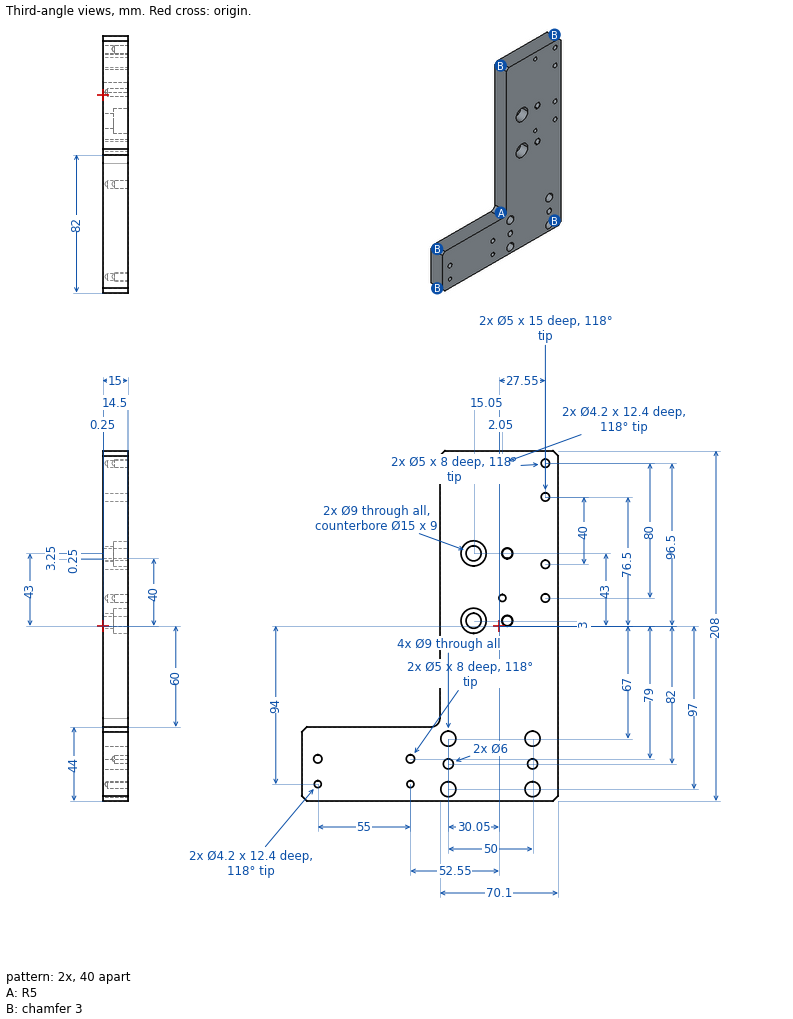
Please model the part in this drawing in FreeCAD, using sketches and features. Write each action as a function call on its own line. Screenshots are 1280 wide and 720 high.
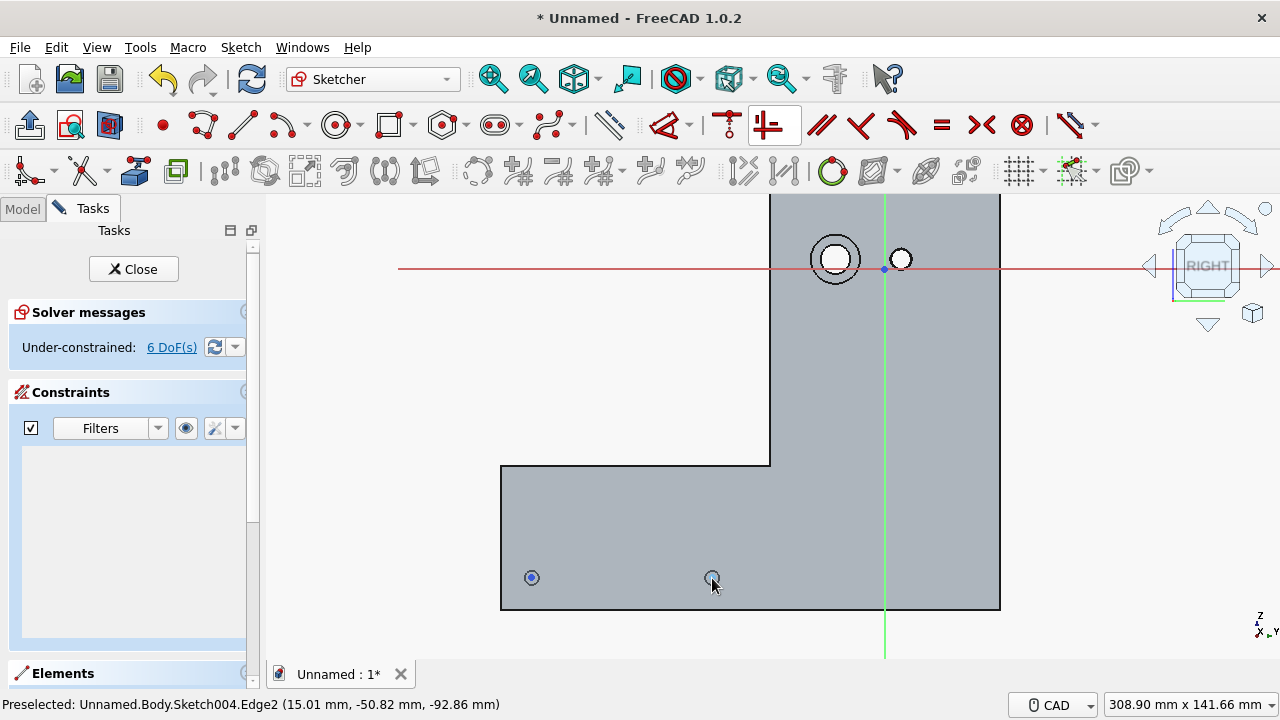
scroll(537, 573, up, 4)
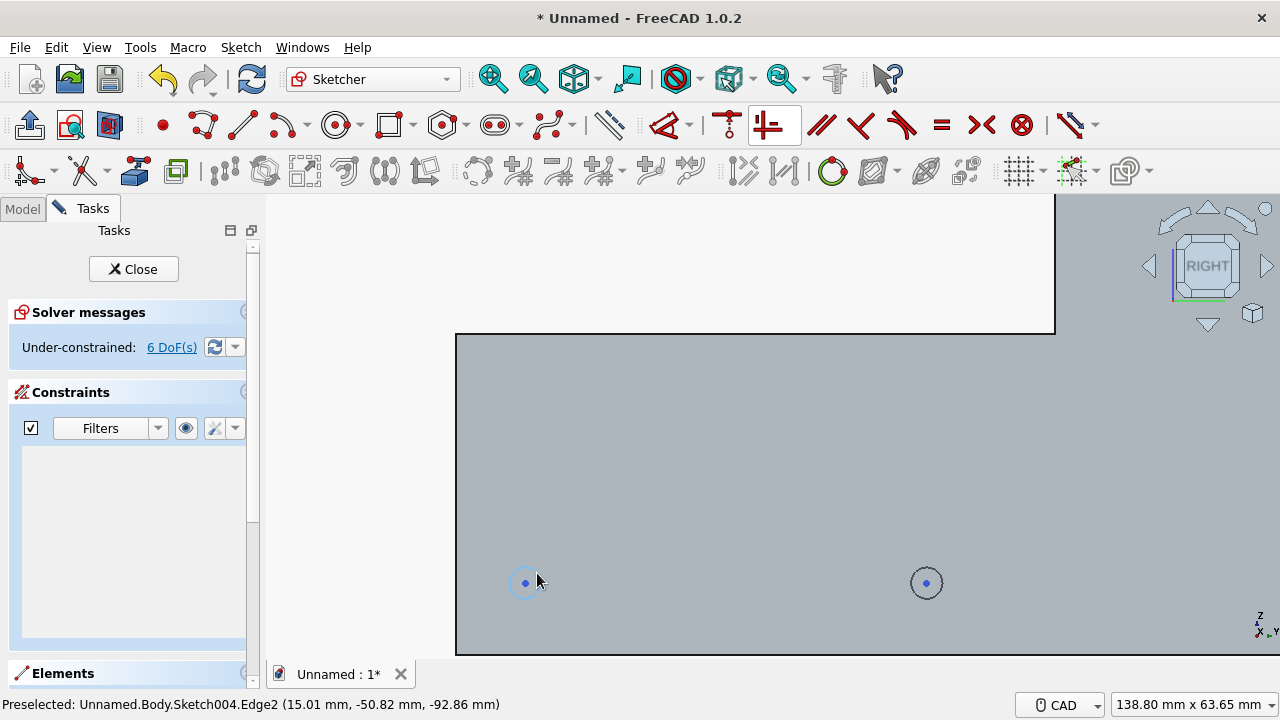
click(536, 572)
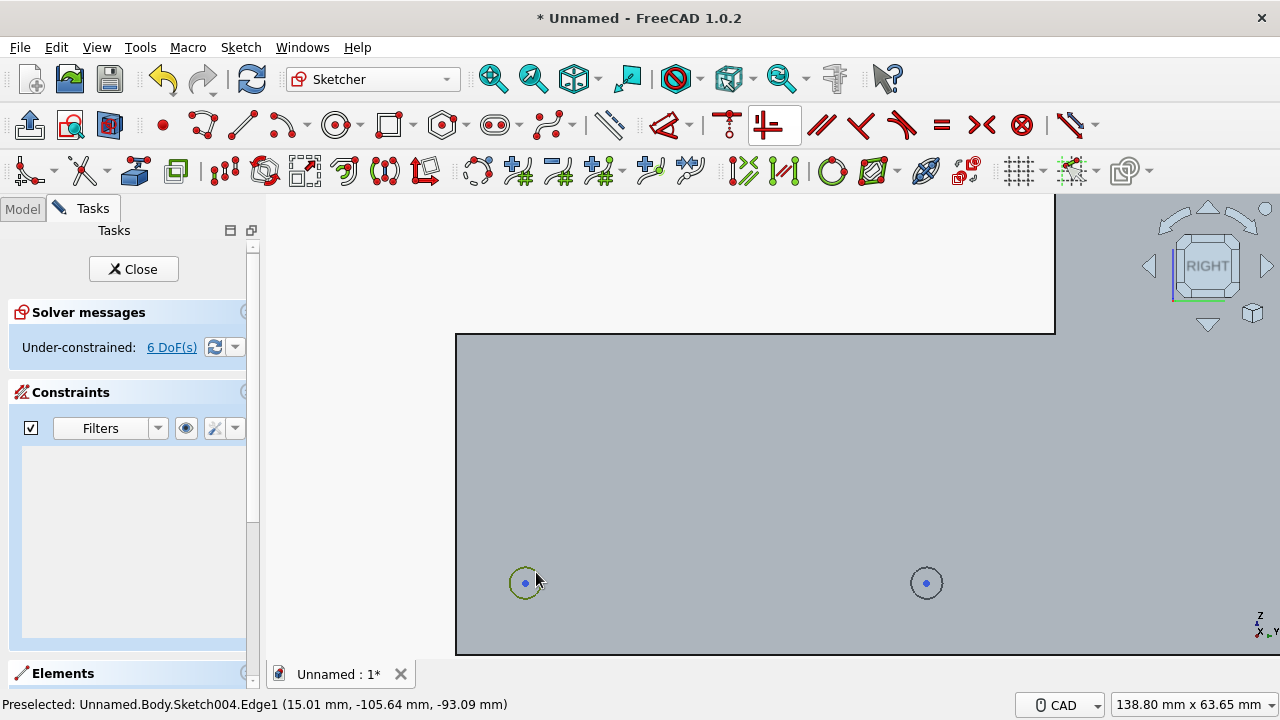
click(938, 572)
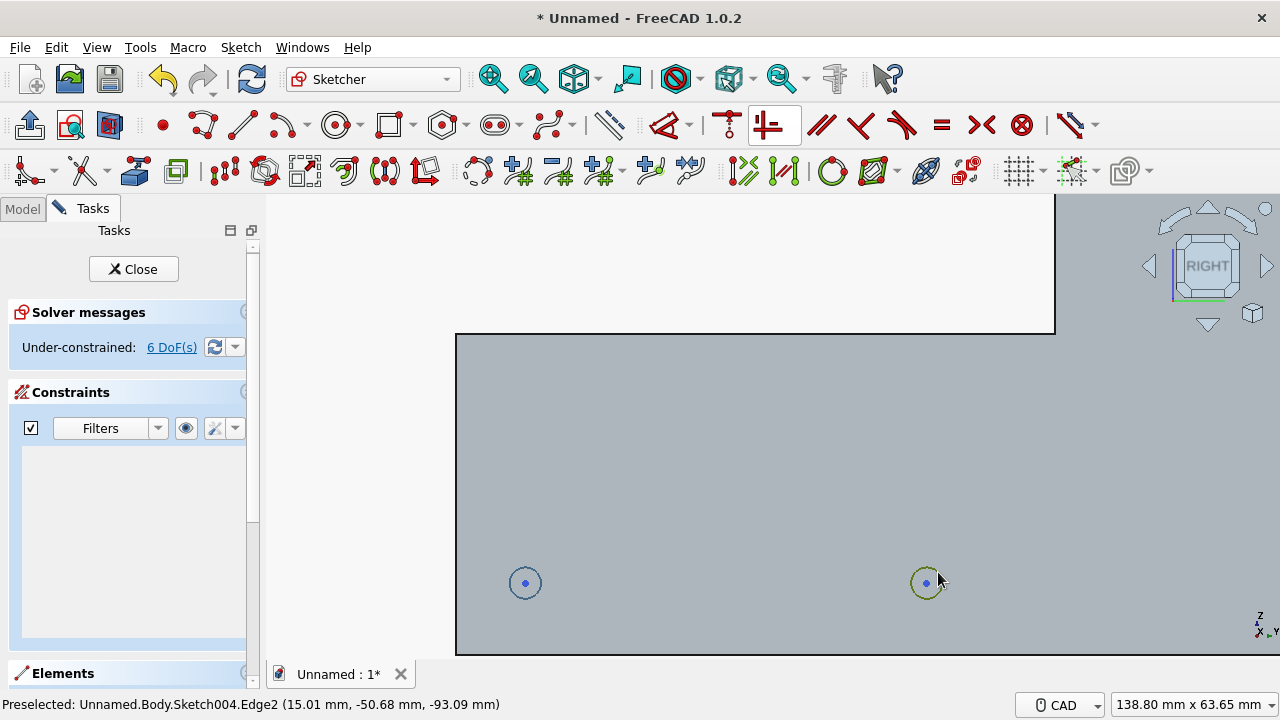
key(e)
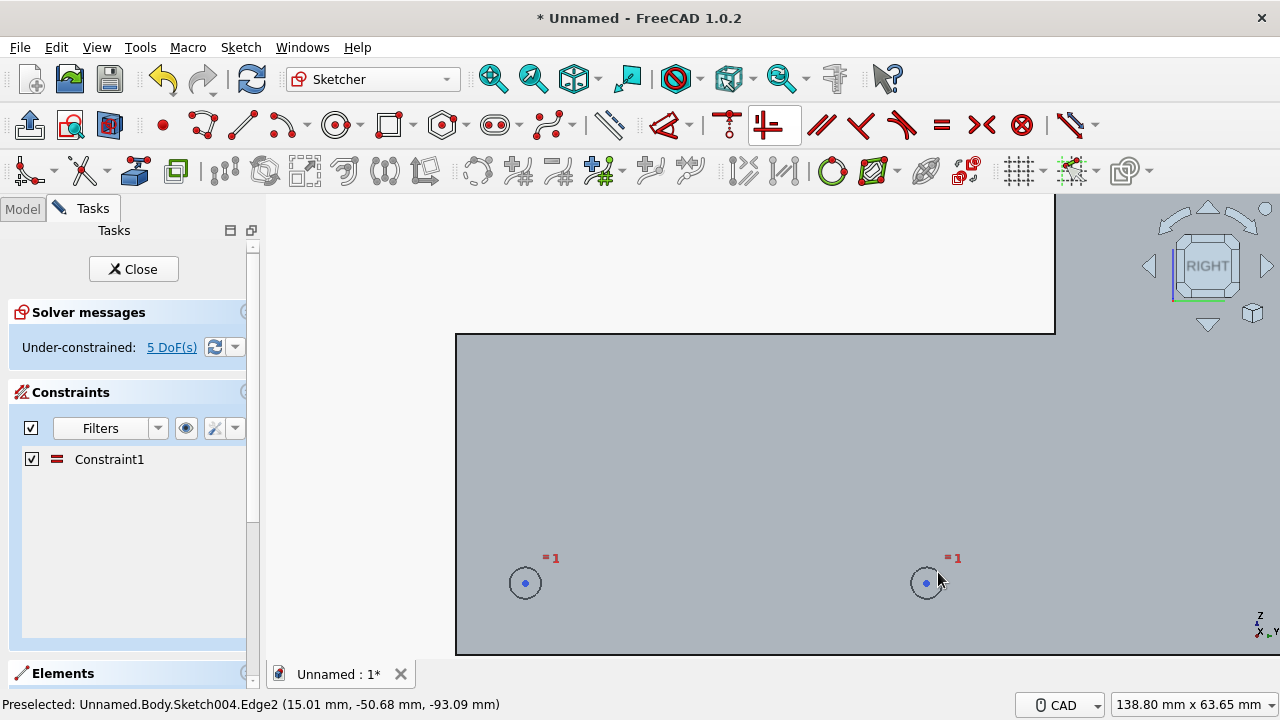
click(525, 583)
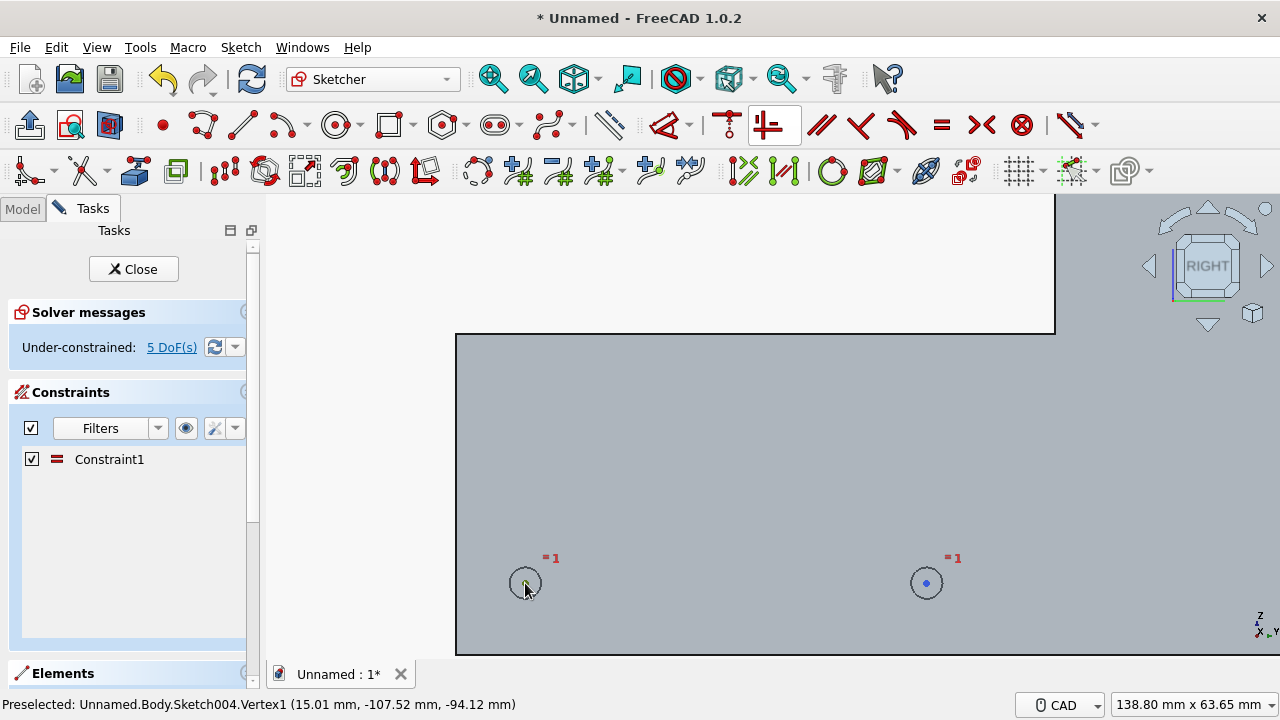
click(927, 583)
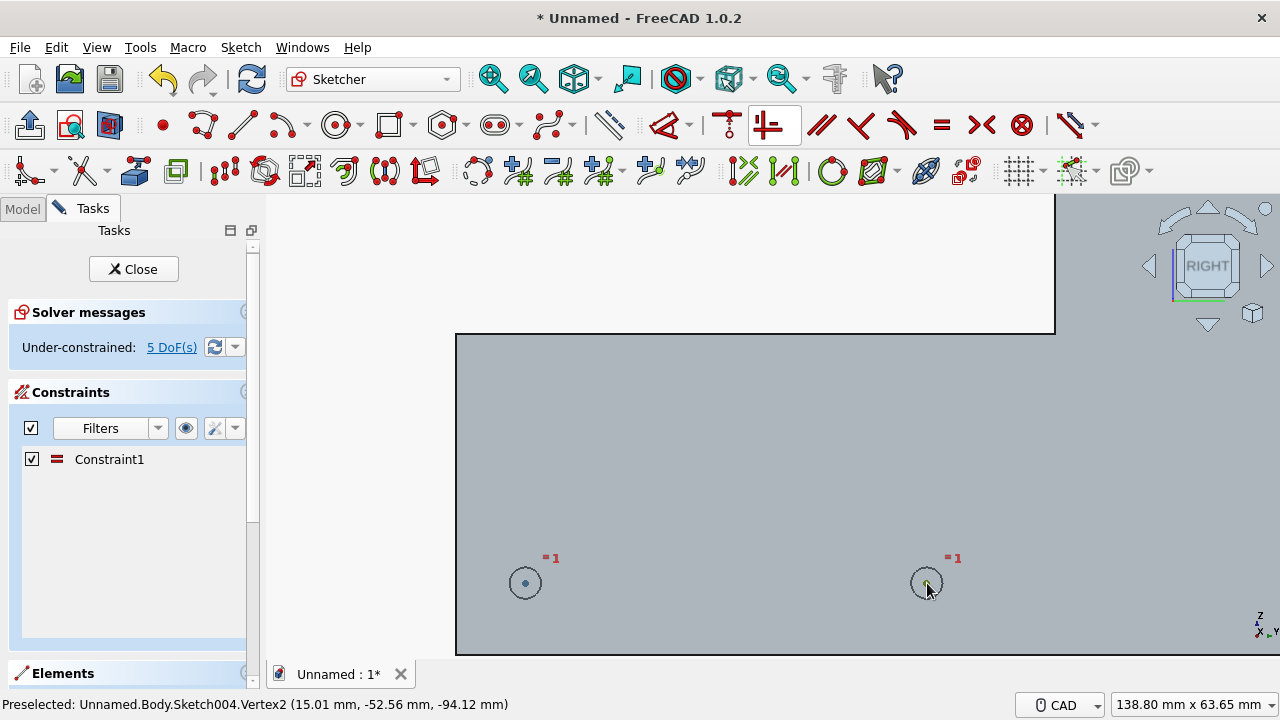
click(796, 126)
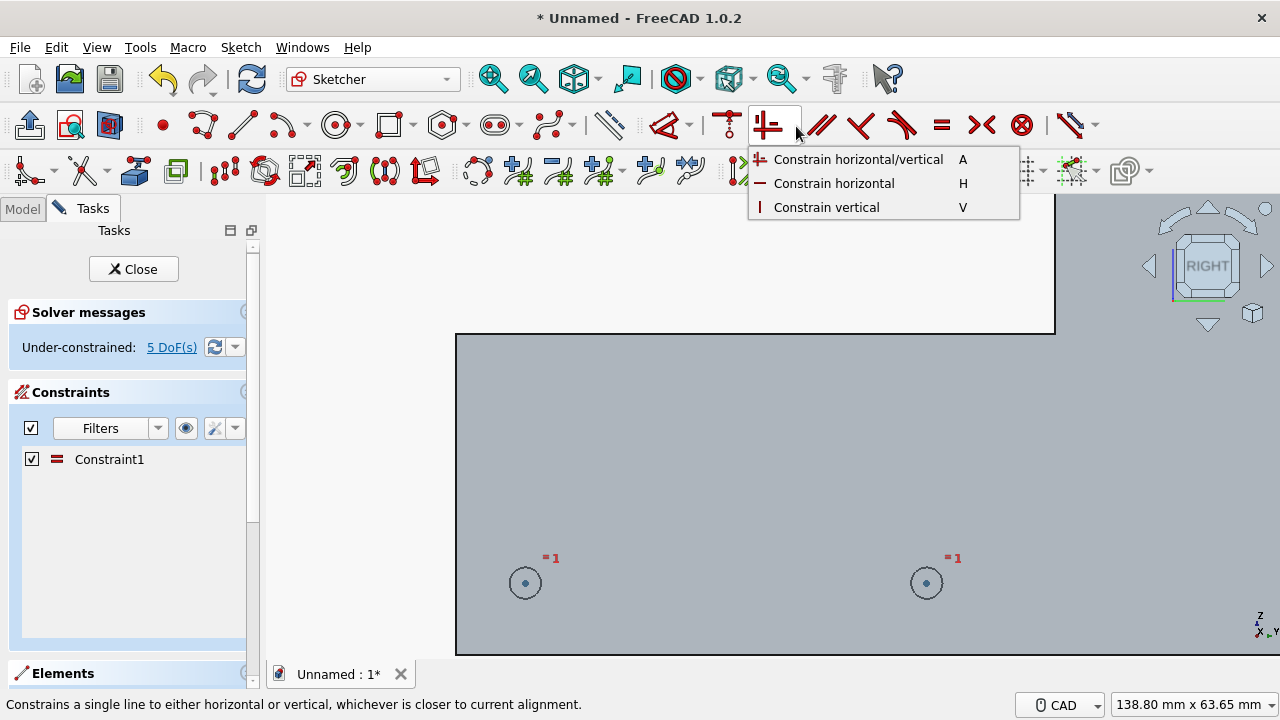
click(884, 183)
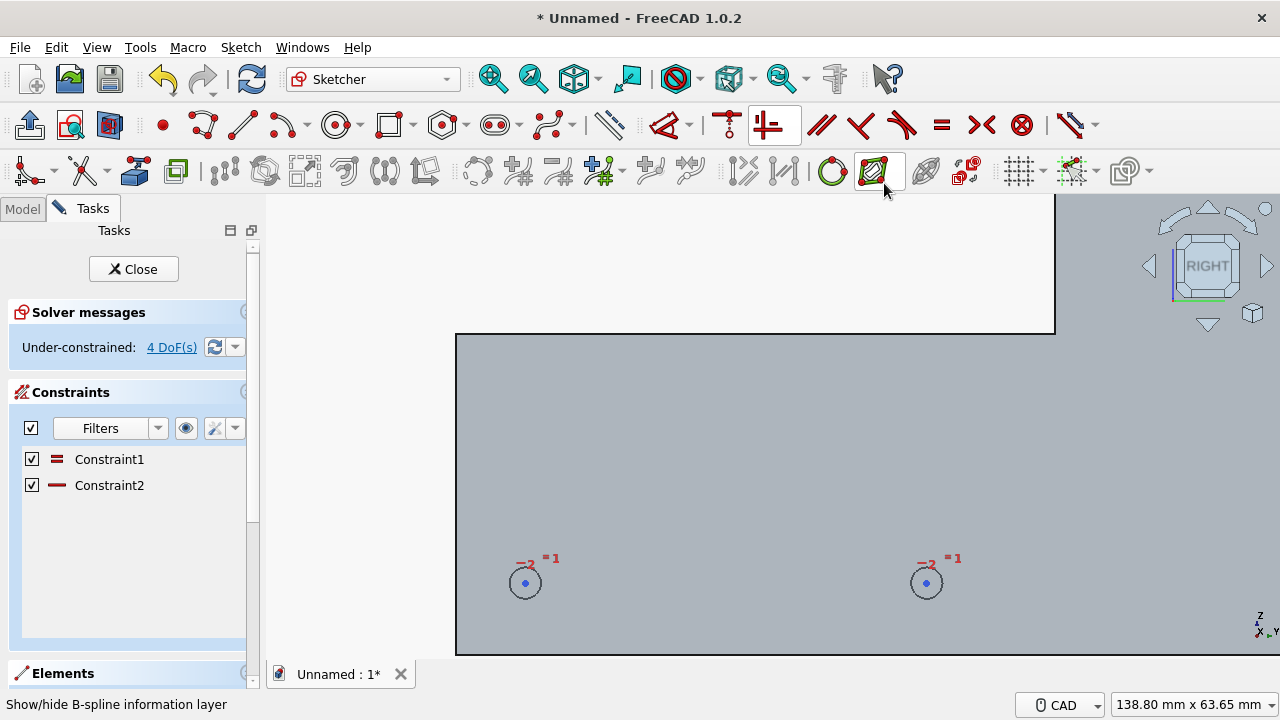
key(d)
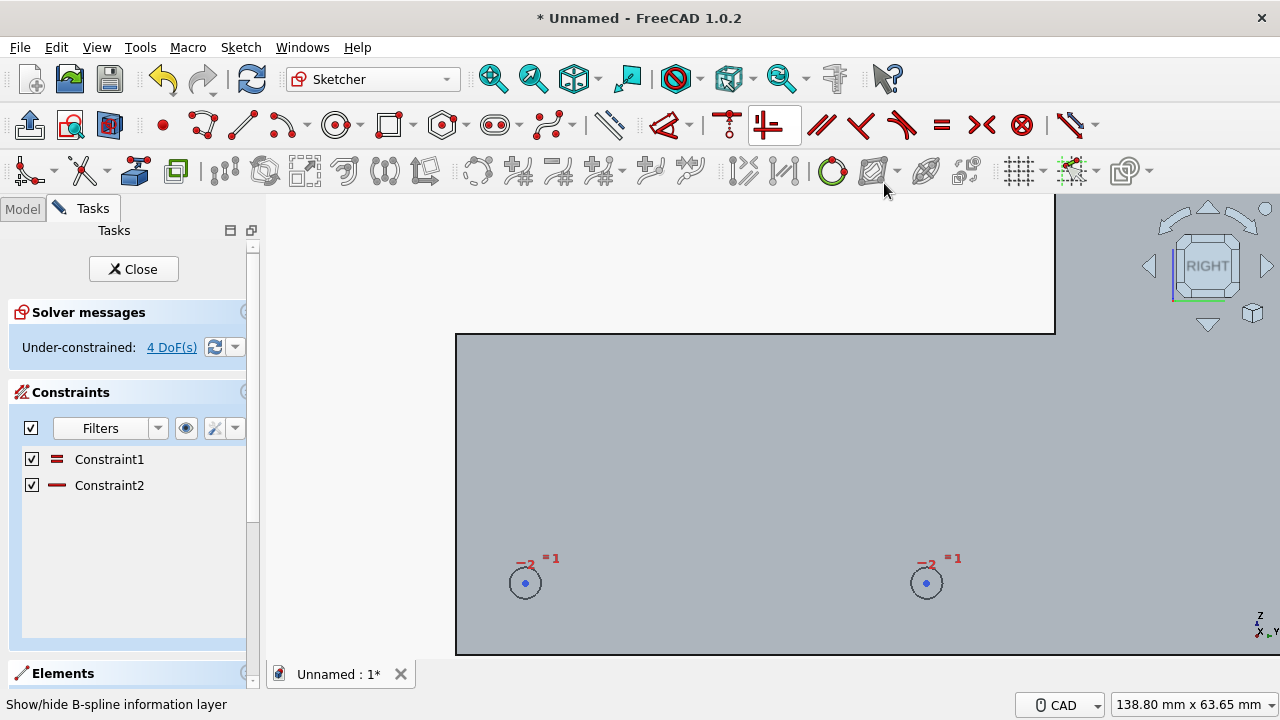
scroll(536, 572, up, 2)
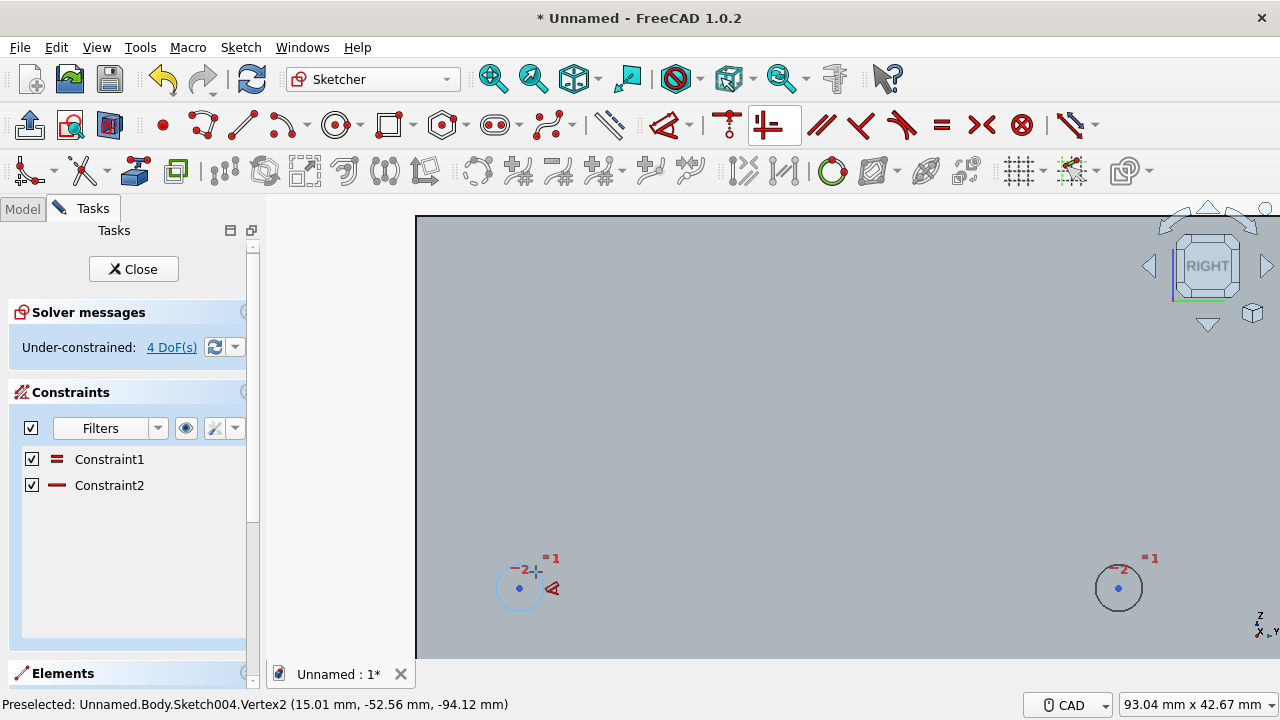
click(536, 572)
click(559, 549)